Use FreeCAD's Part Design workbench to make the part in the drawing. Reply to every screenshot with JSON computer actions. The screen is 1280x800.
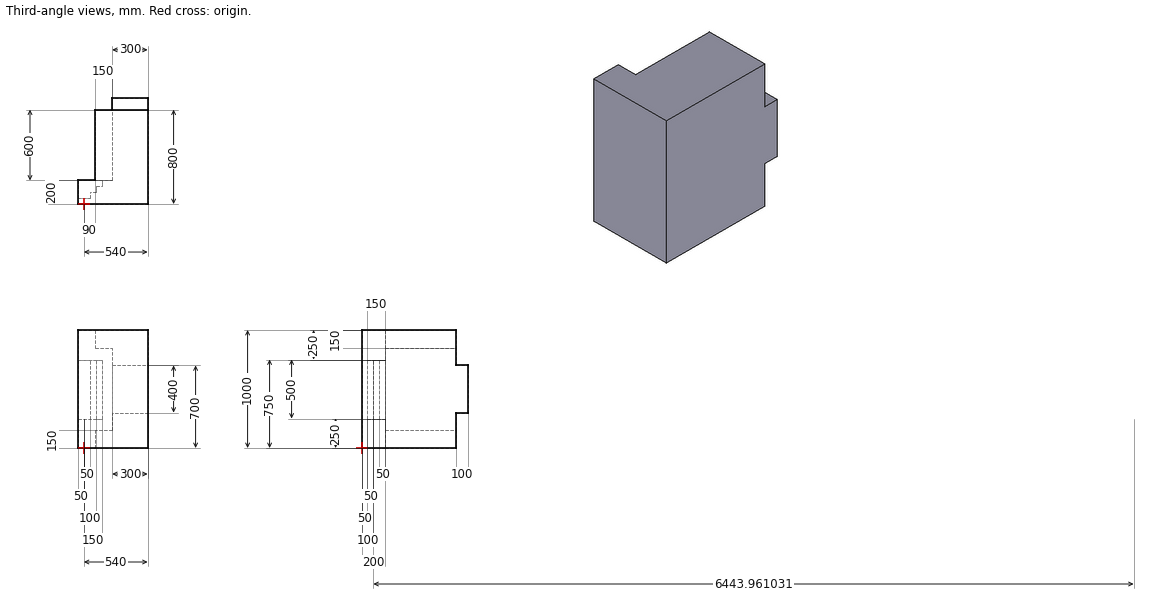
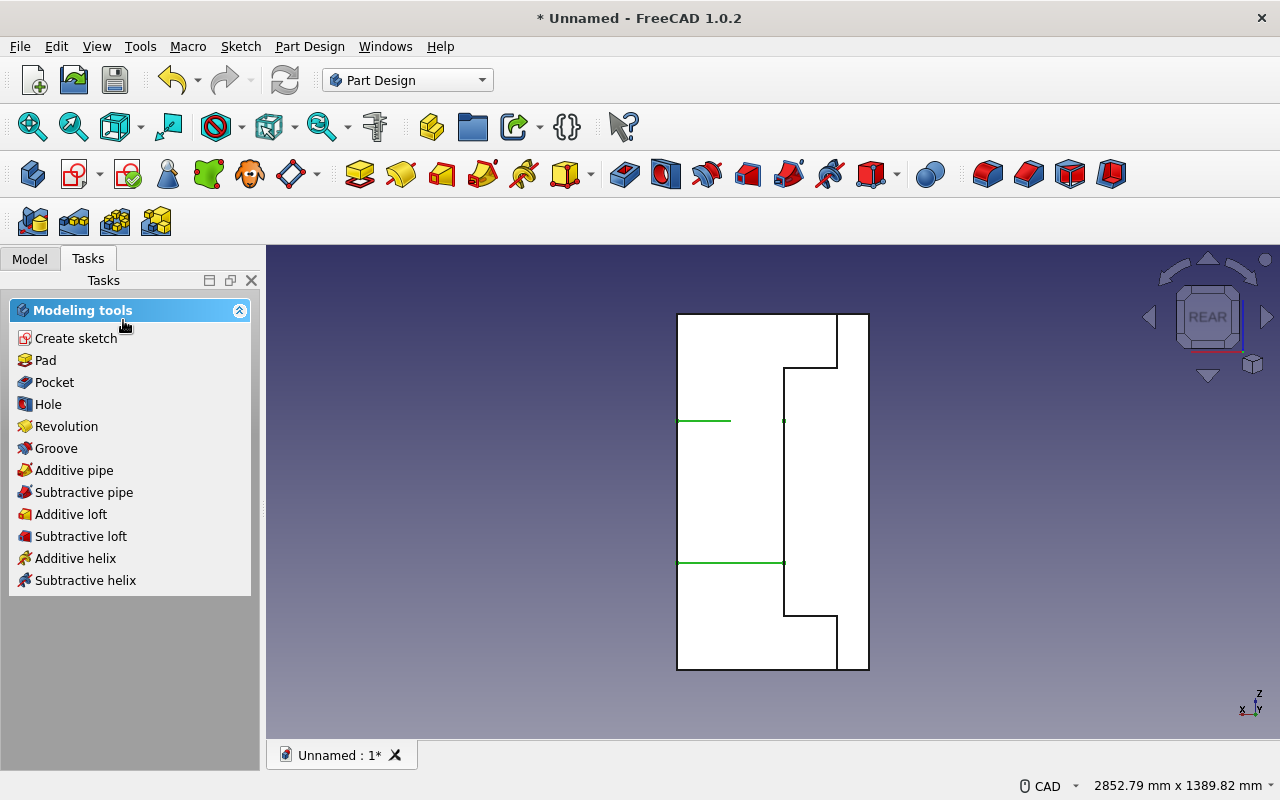
{"action": "left_click", "coordinate": [360, 174]}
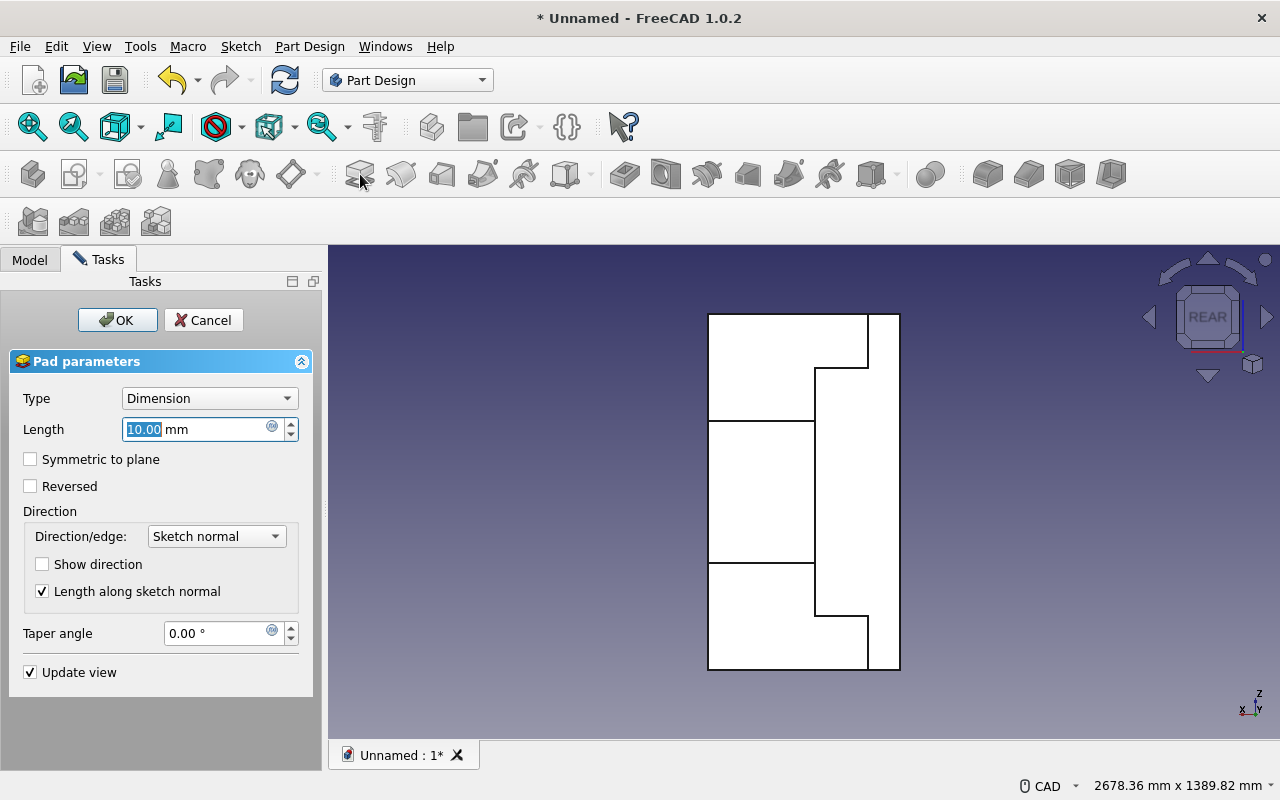
{"action": "type", "text": "100"}
{"action": "key", "text": "Tab"}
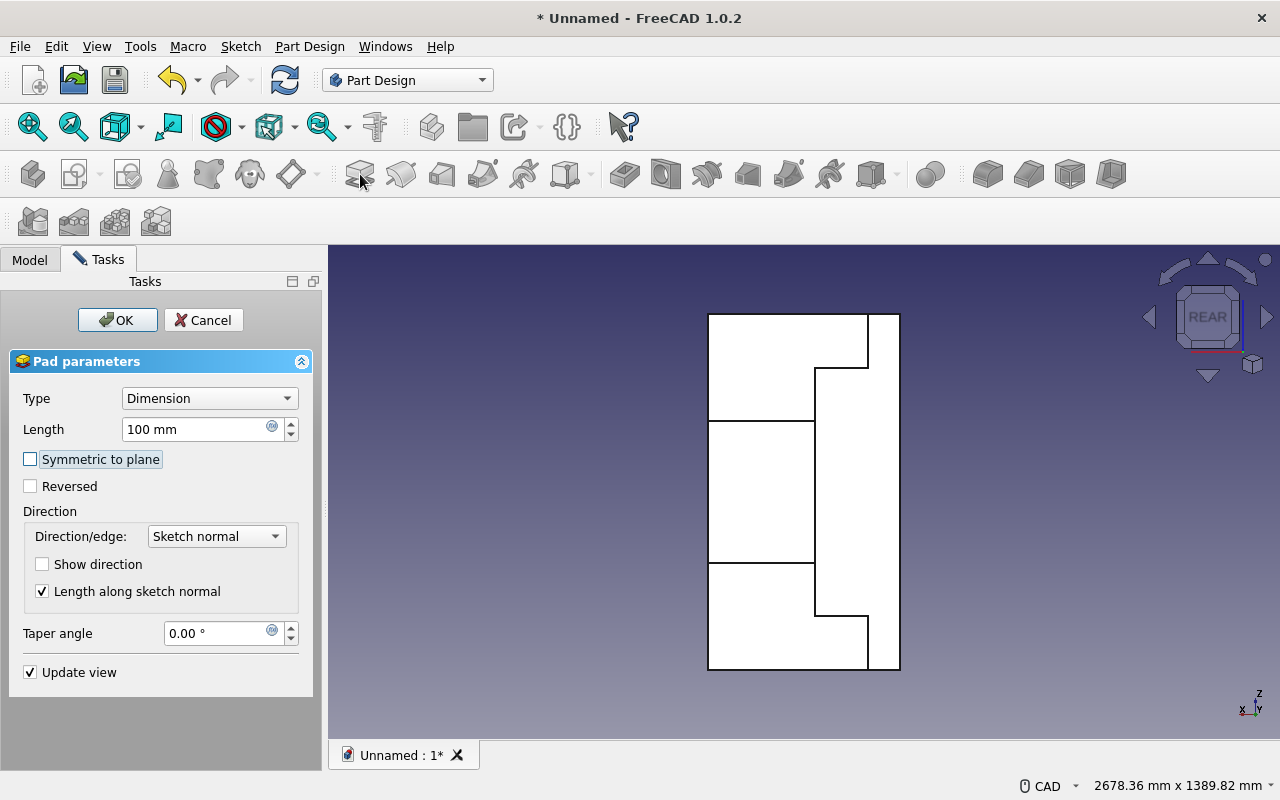
{"action": "left_click", "coordinate": [118, 320]}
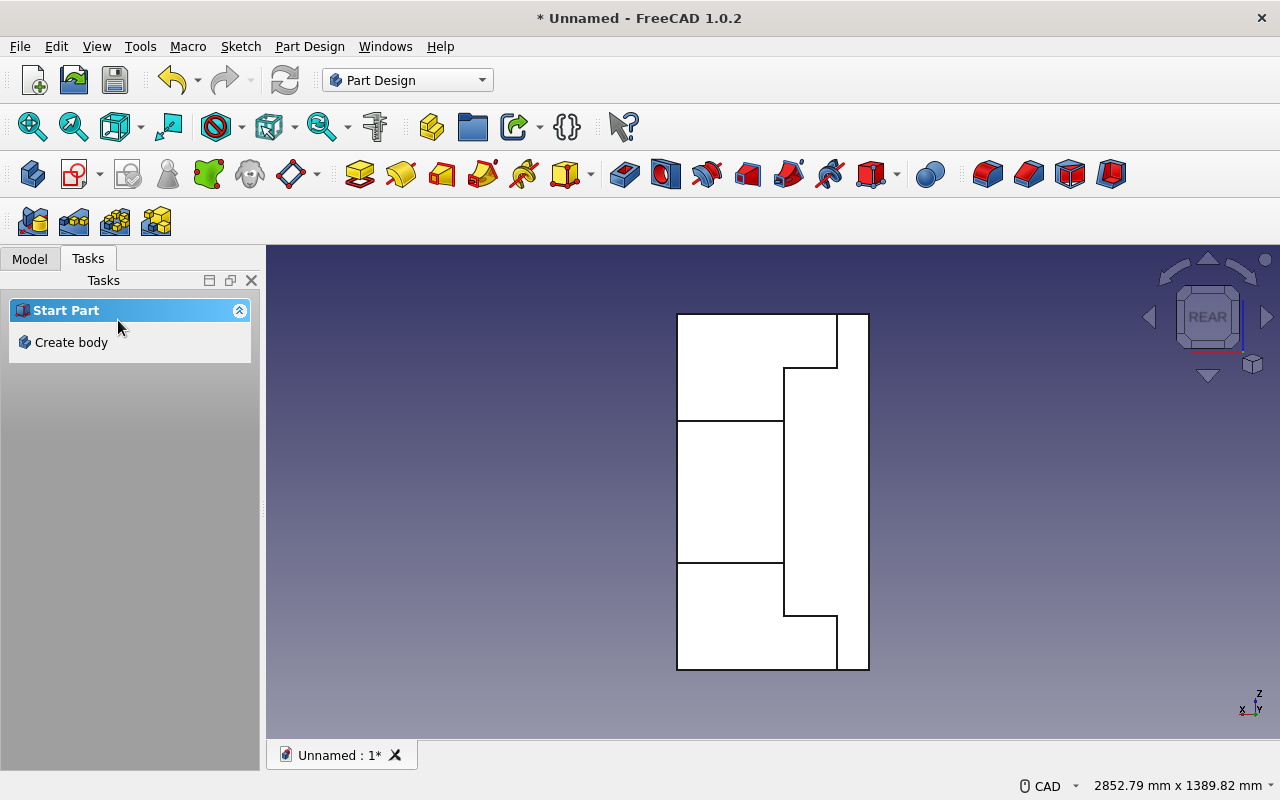
{"action": "key", "text": "6"}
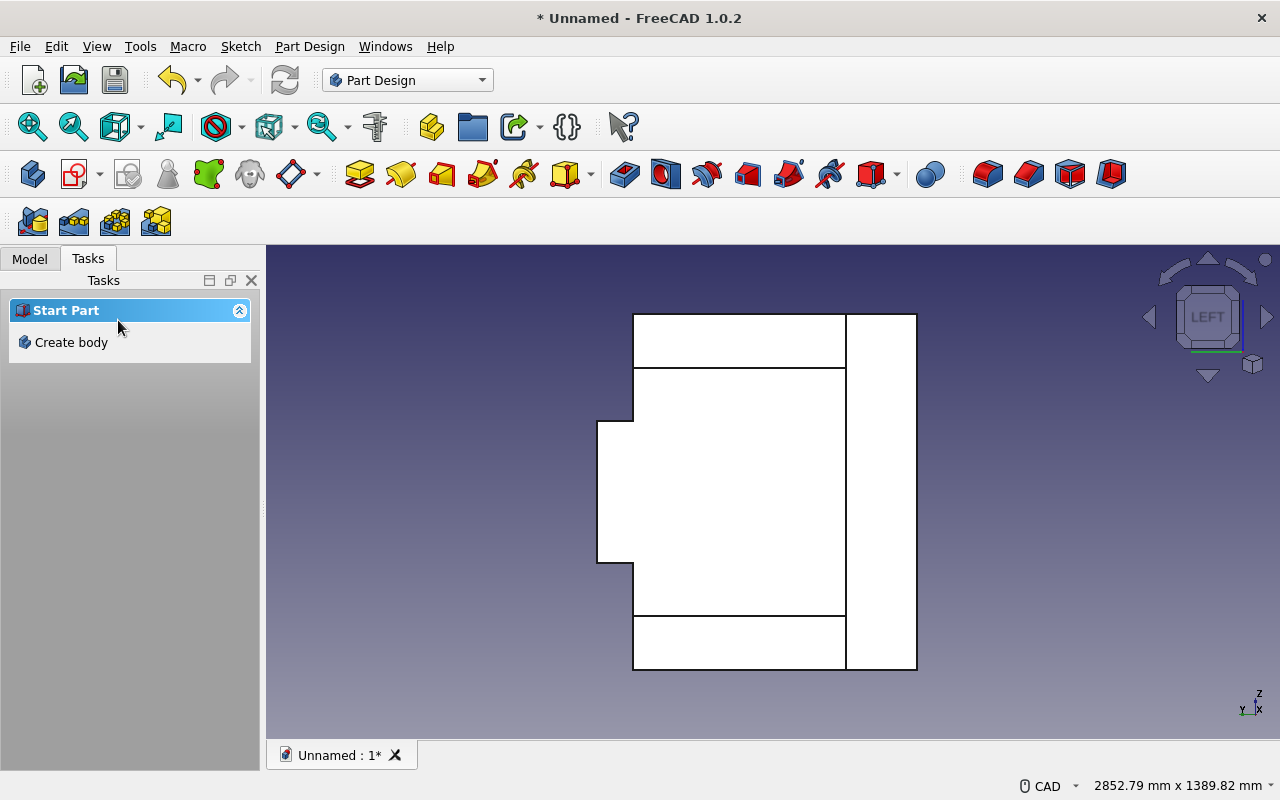
{"action": "left_click", "coordinate": [881, 389]}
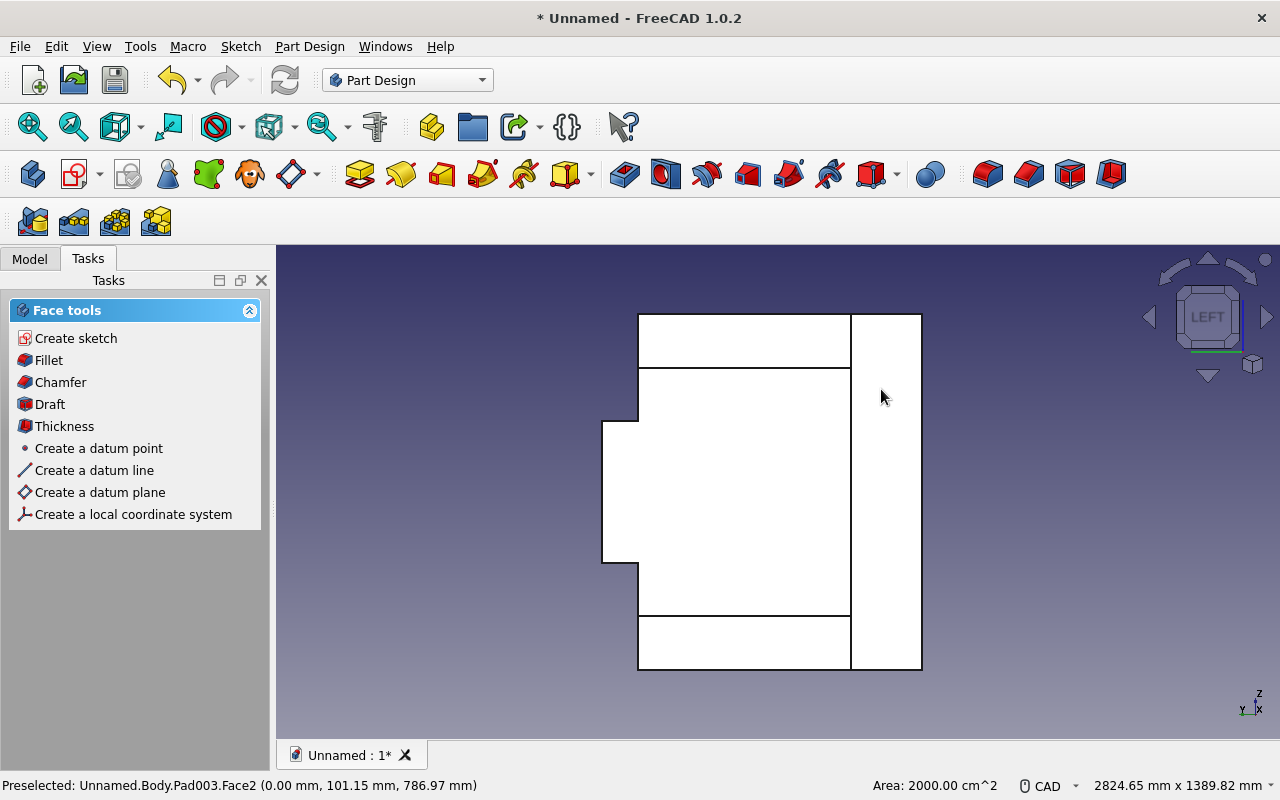
{"action": "left_click", "coordinate": [74, 174]}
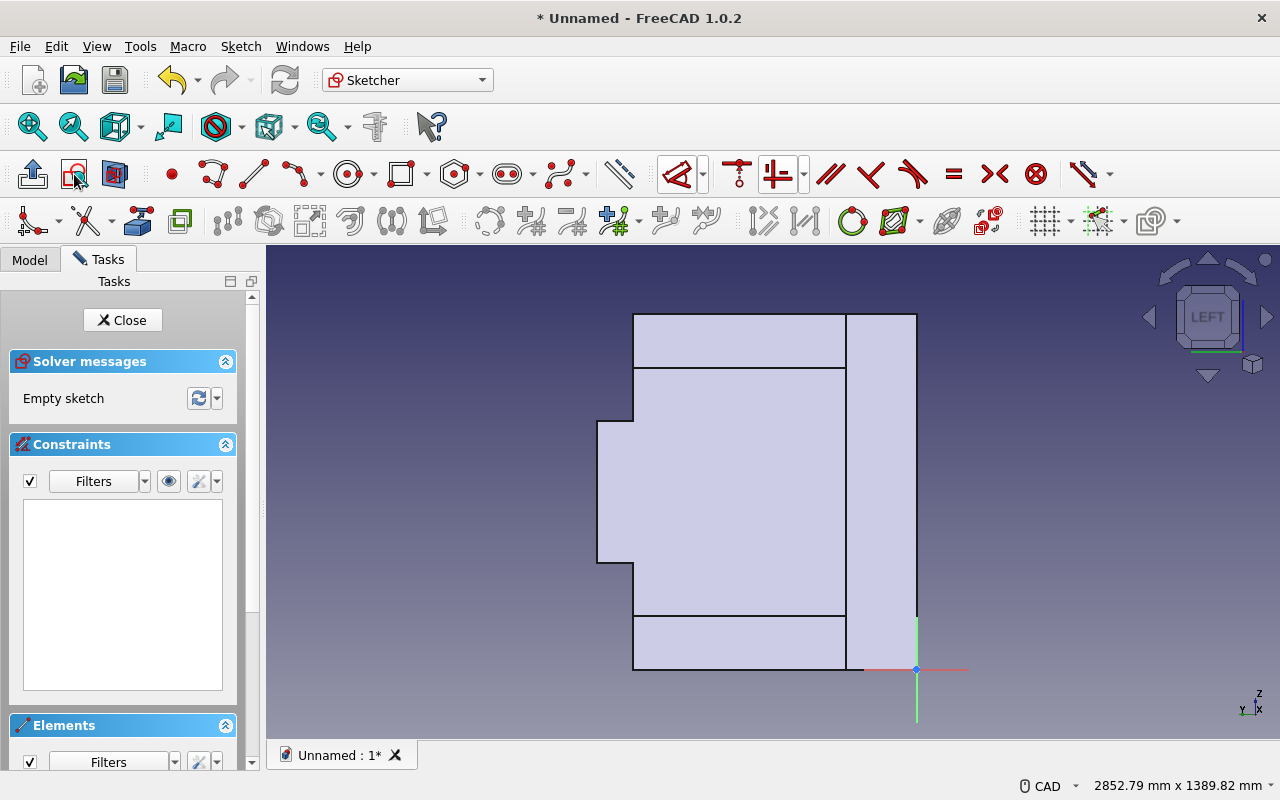
{"action": "left_click", "coordinate": [400, 174]}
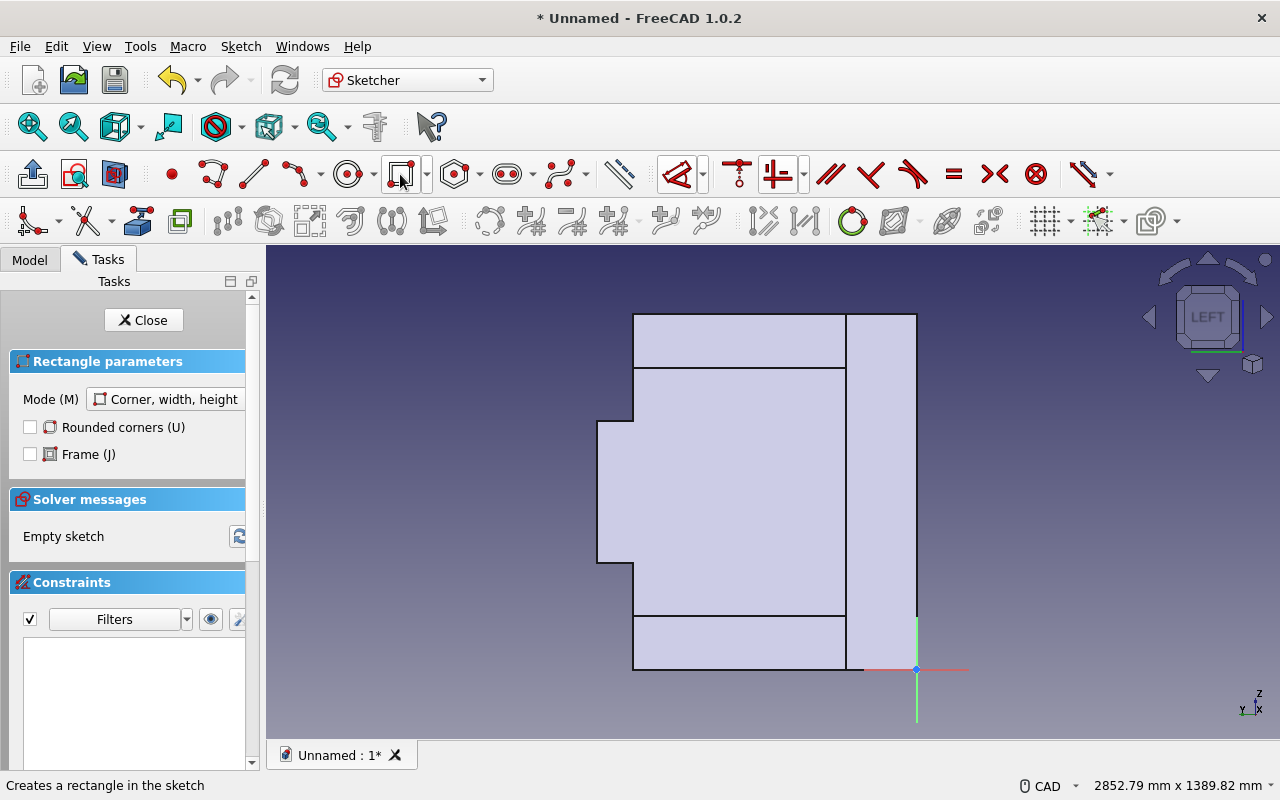
{"action": "left_click", "coordinate": [846, 403]}
{"action": "left_click", "coordinate": [864, 581]}
{"action": "key", "text": "Escape"}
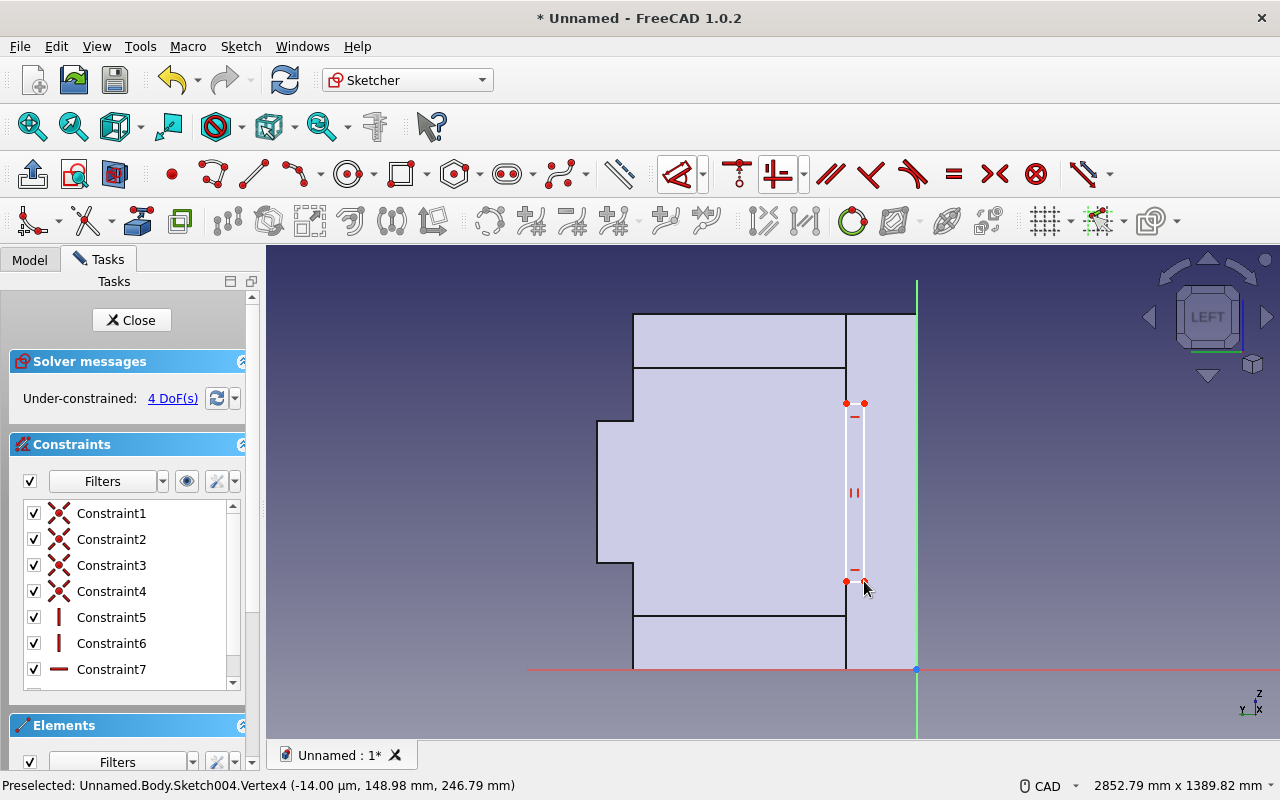
{"action": "scroll", "coordinate": [855, 582], "scroll_direction": "up", "scroll_amount": 5}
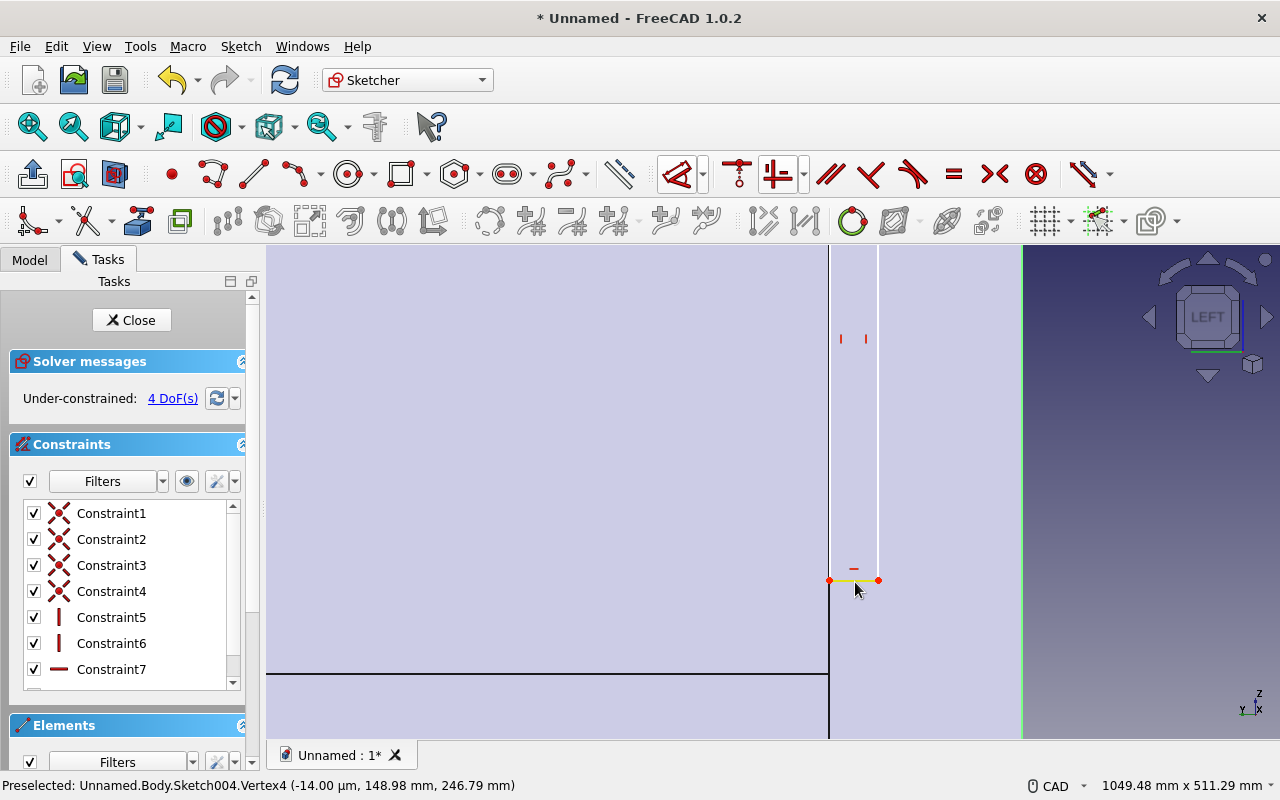
{"action": "left_click", "coordinate": [854, 581]}